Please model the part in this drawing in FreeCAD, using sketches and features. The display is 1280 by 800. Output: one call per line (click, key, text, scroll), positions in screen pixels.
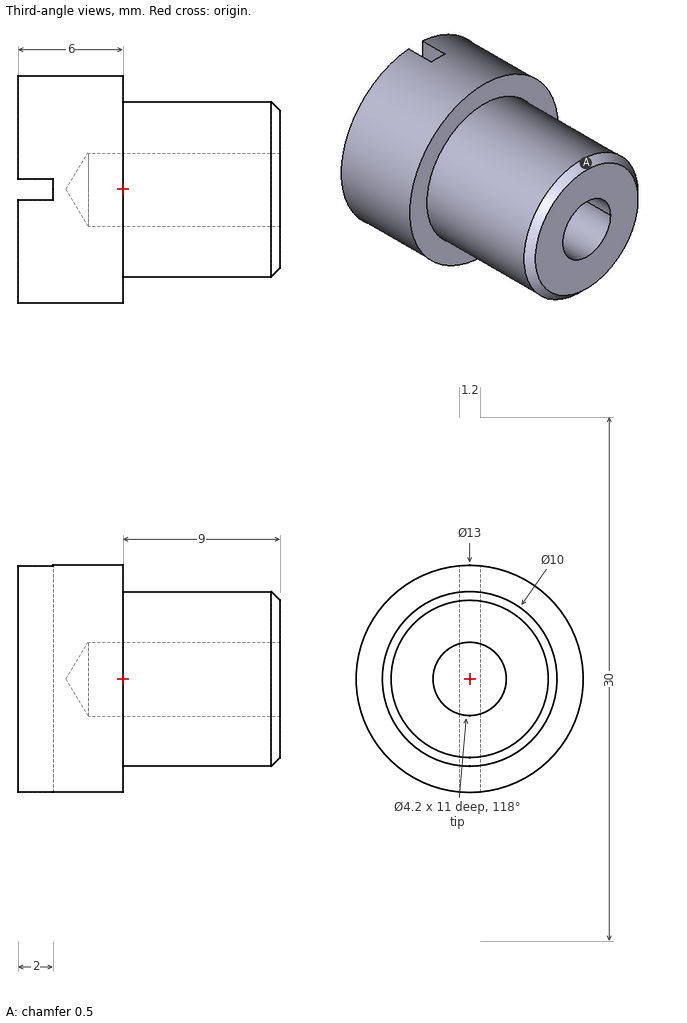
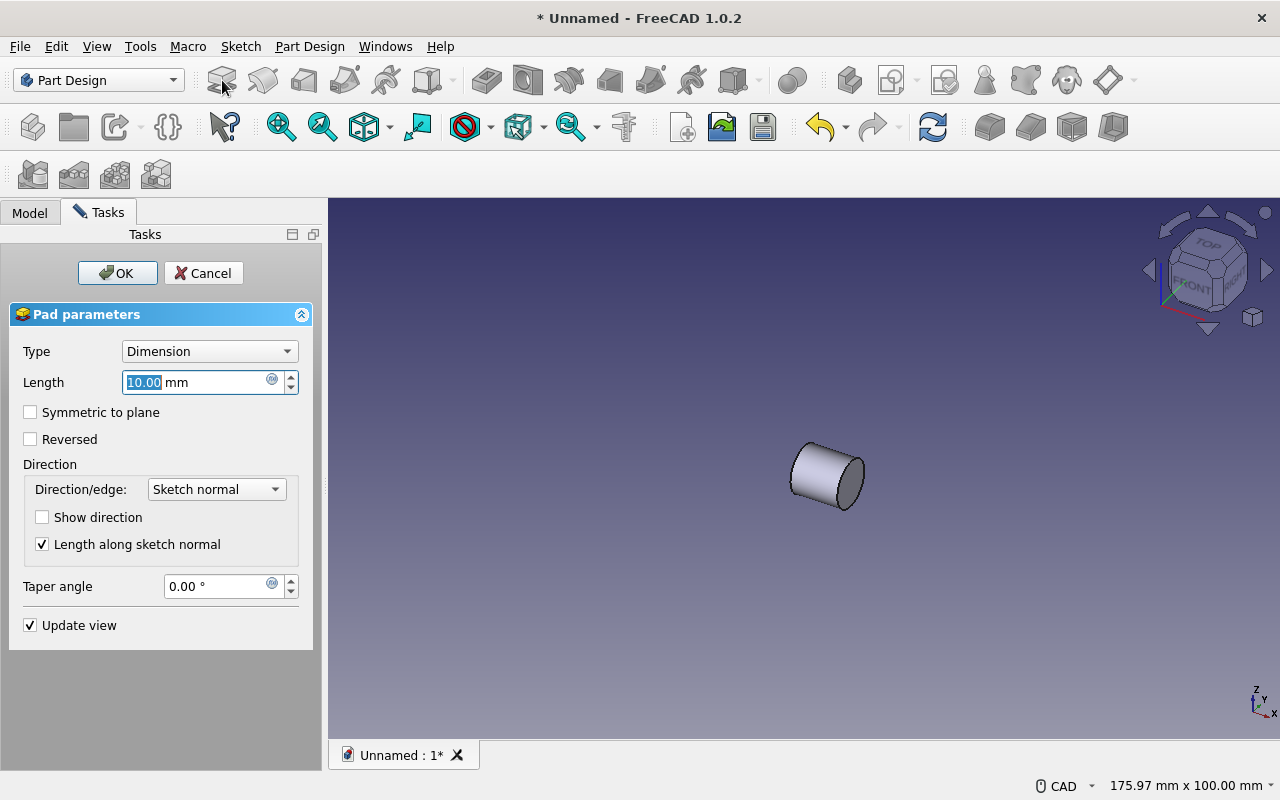
text(9)
key(Tab)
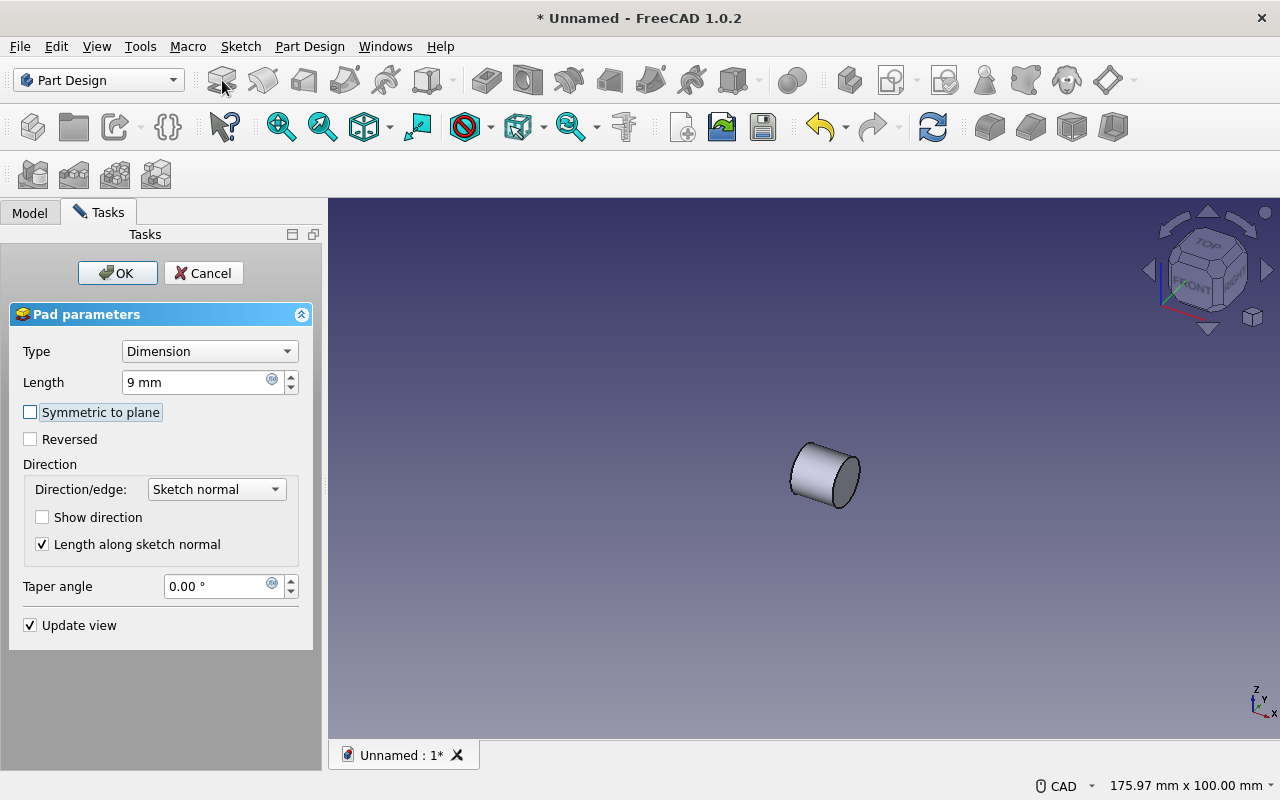
click(118, 273)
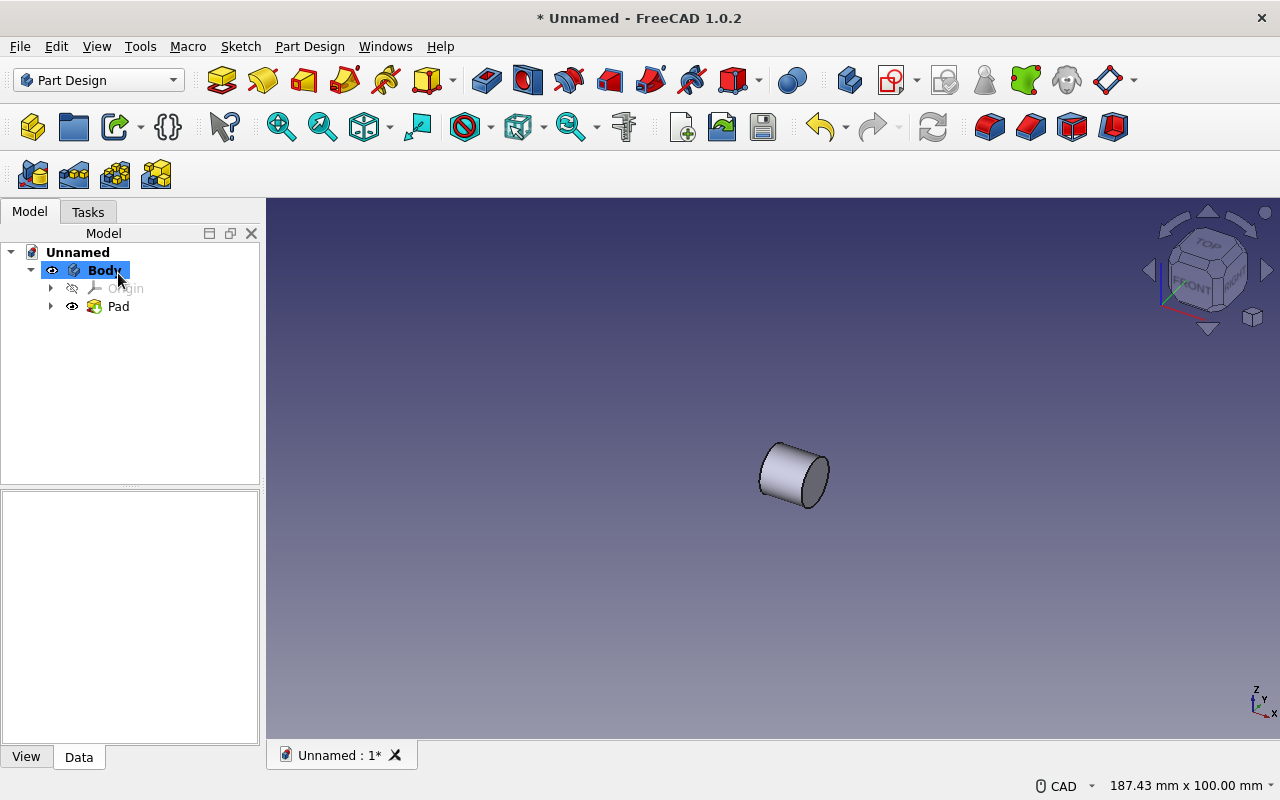
click(282, 128)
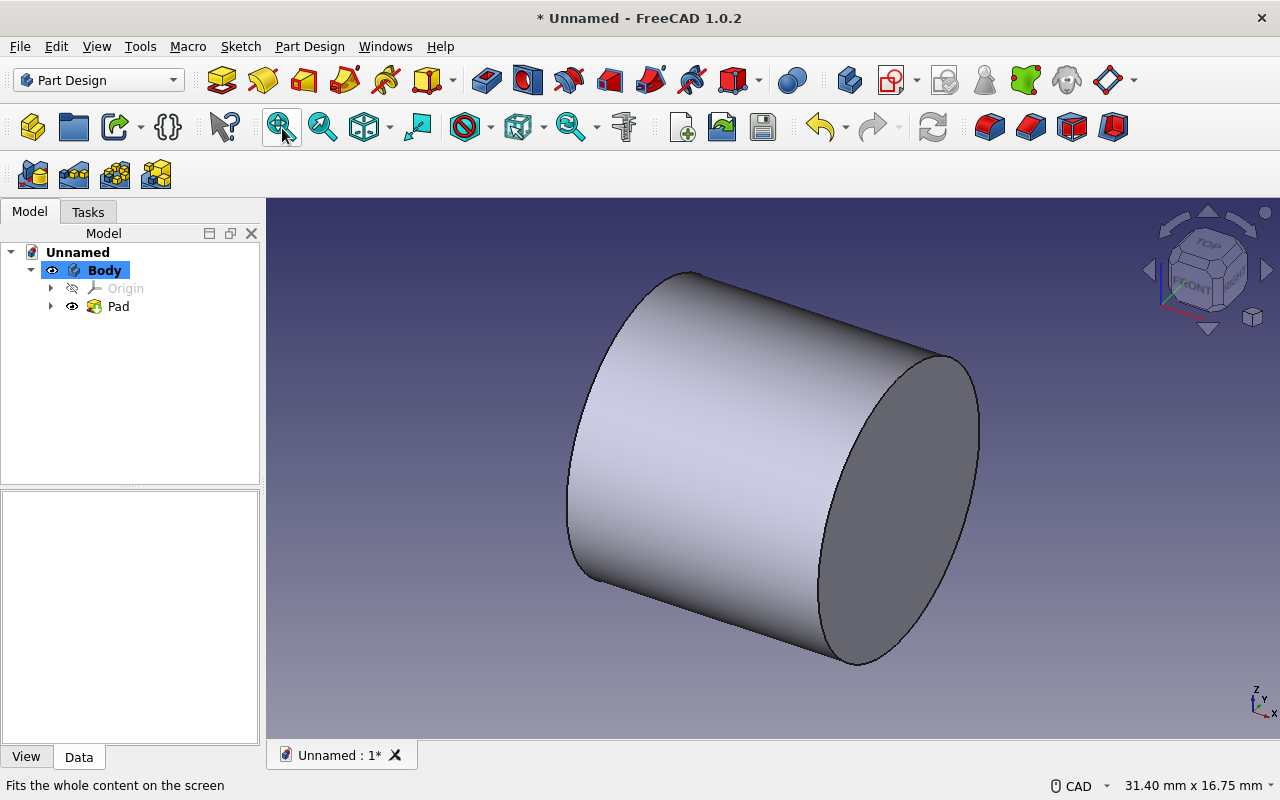
key(6)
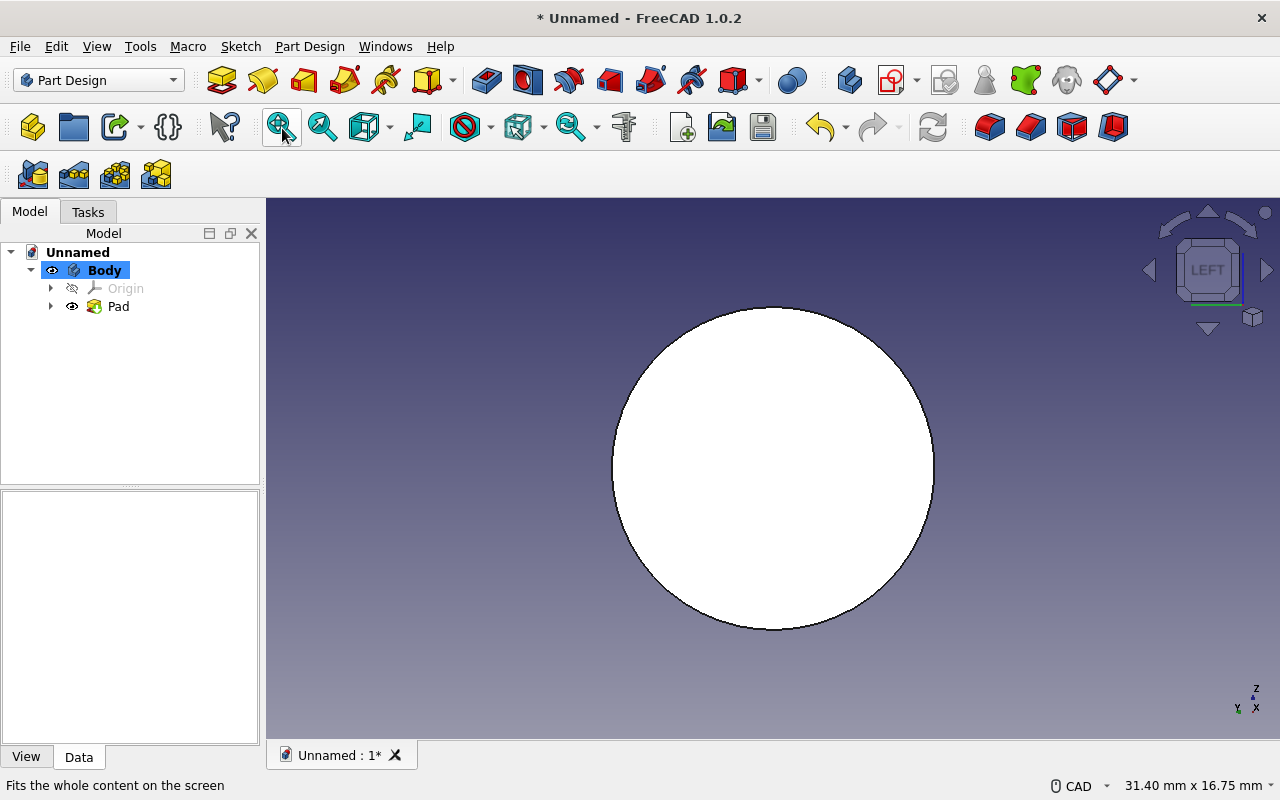
click(773, 467)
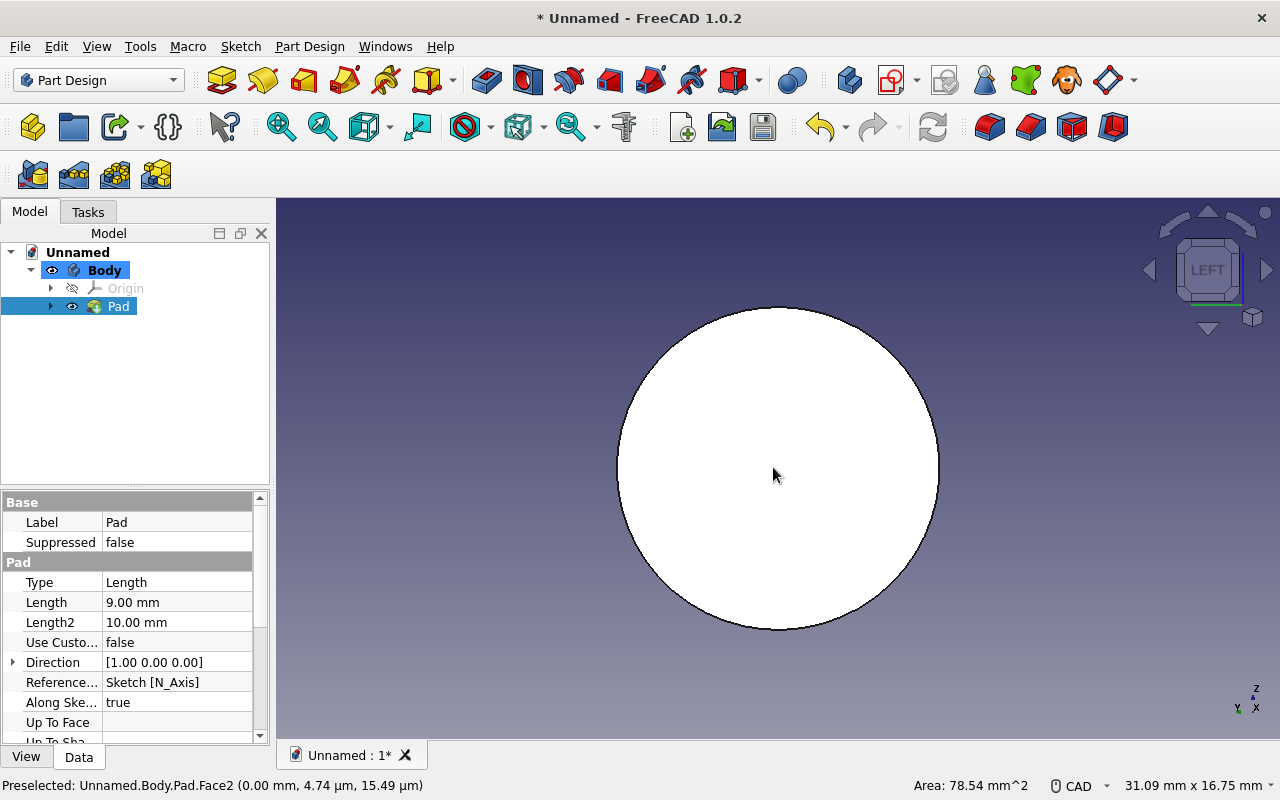
click(890, 80)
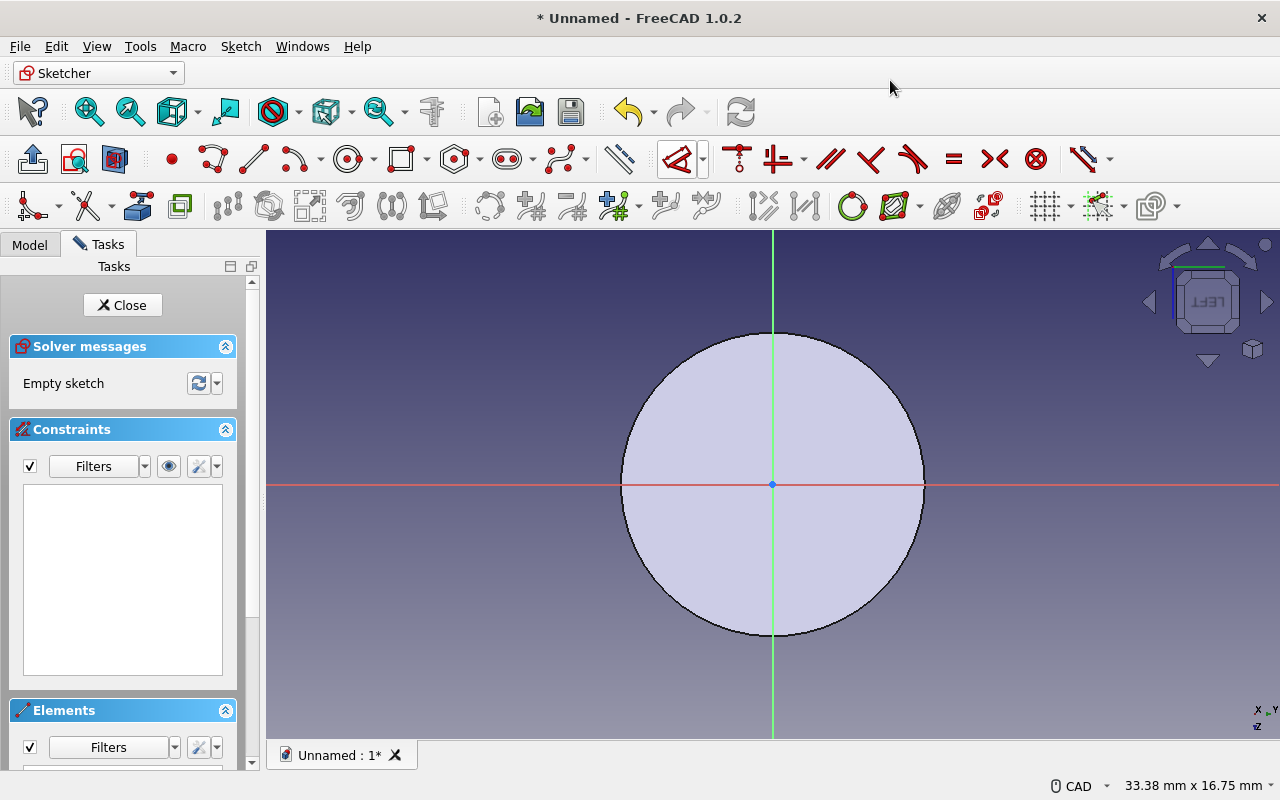
click(348, 160)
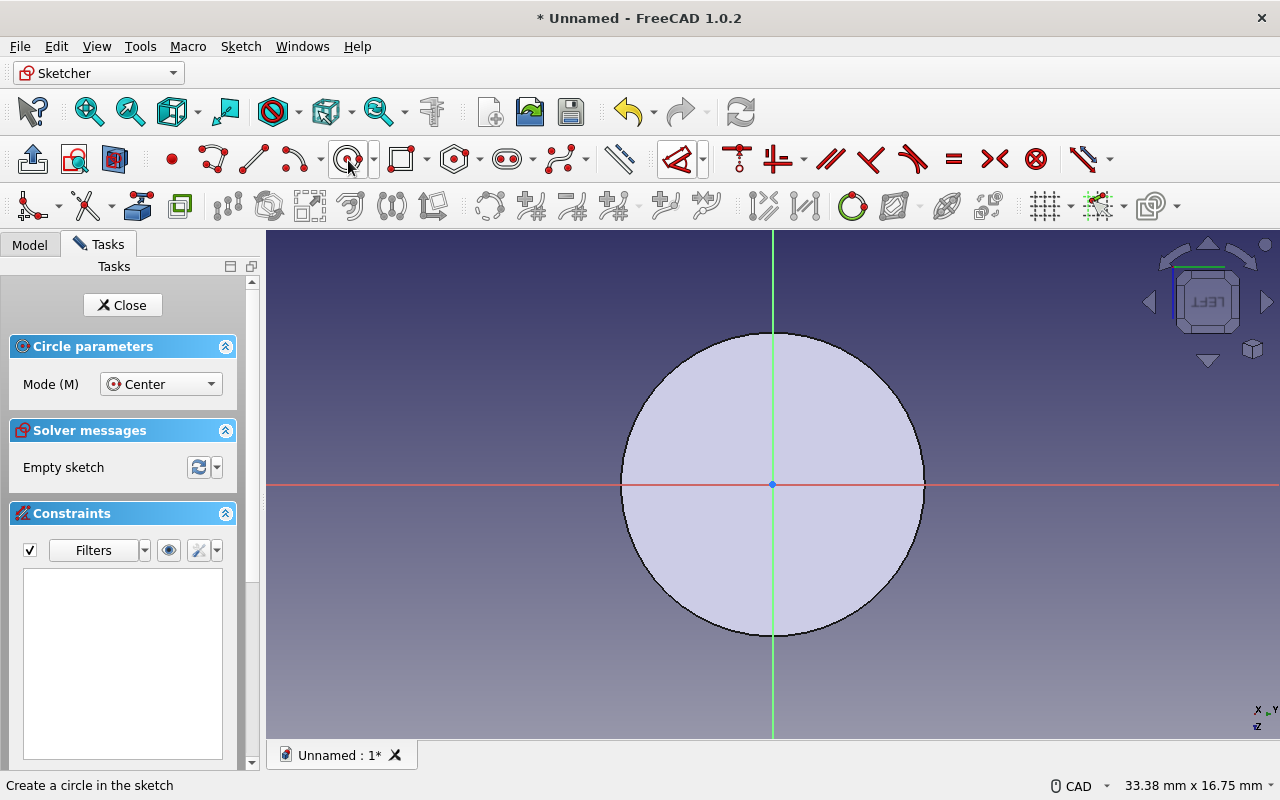
click(773, 484)
move(912, 345)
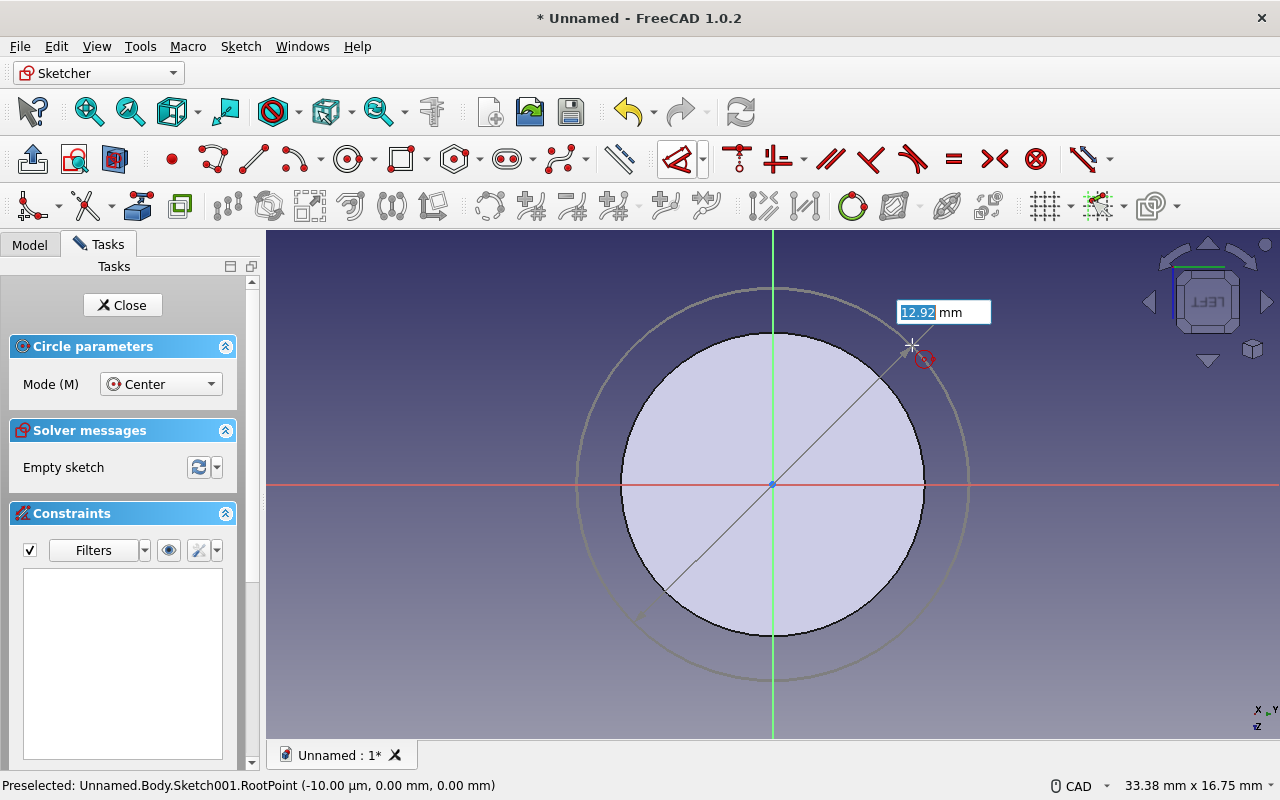
text(13)
key(Return)
key(Escape)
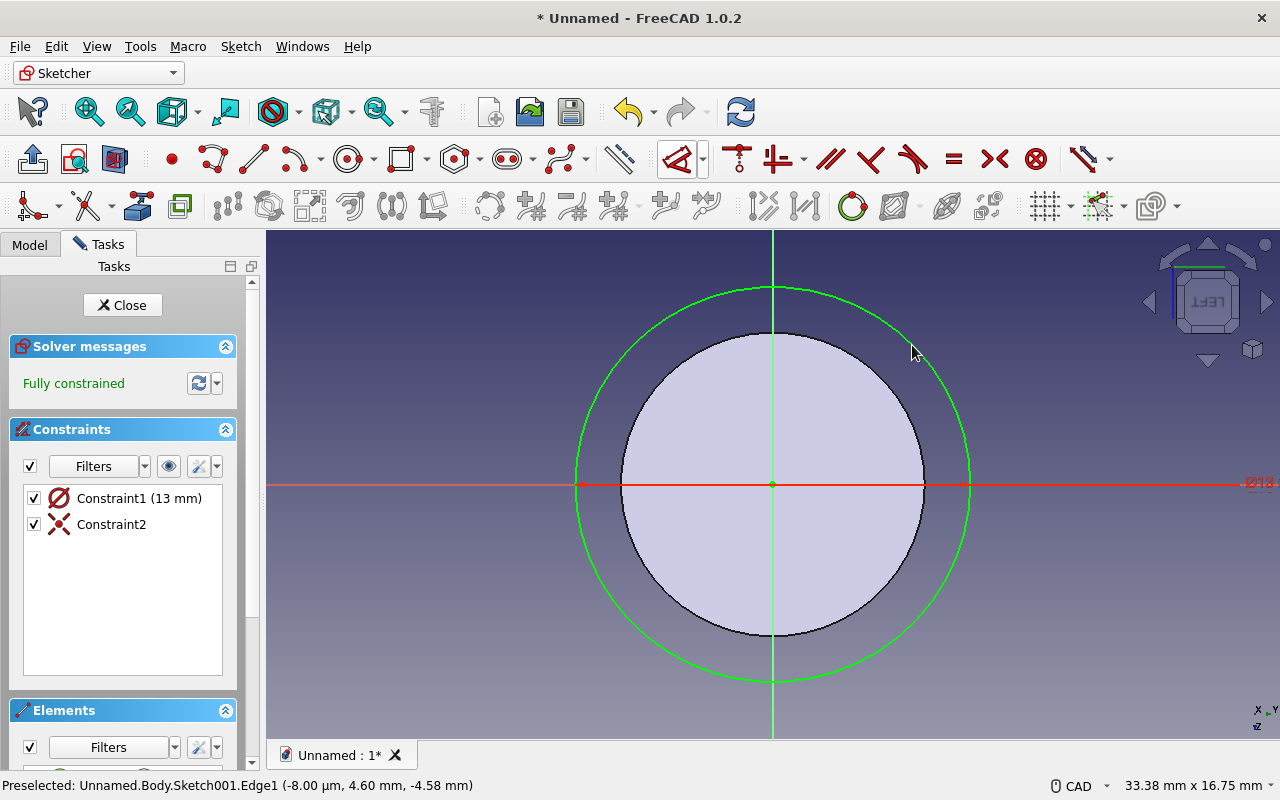
click(123, 305)